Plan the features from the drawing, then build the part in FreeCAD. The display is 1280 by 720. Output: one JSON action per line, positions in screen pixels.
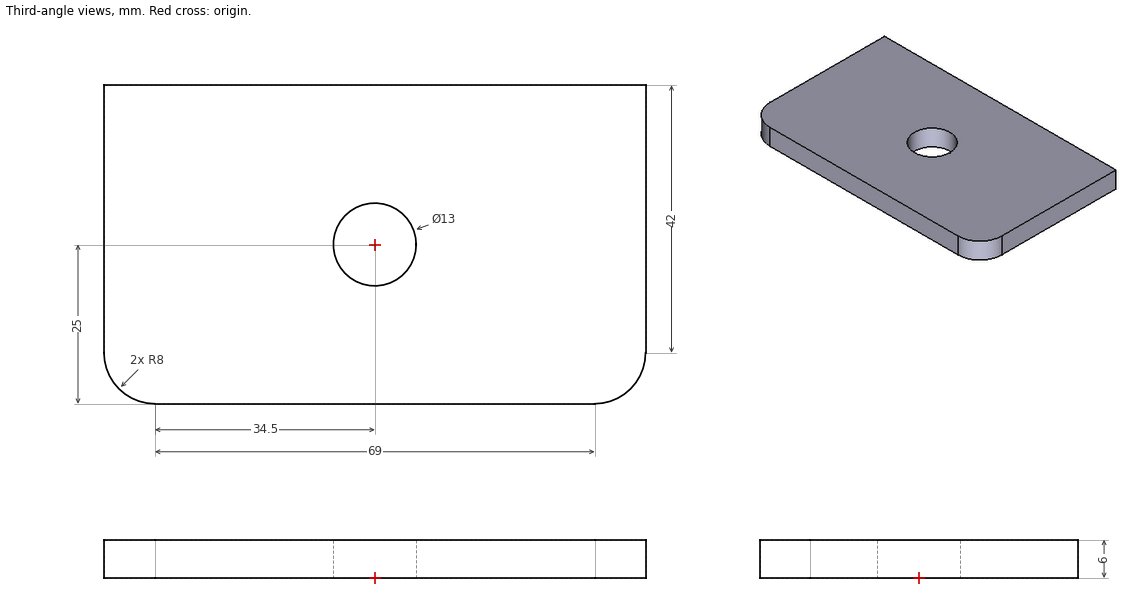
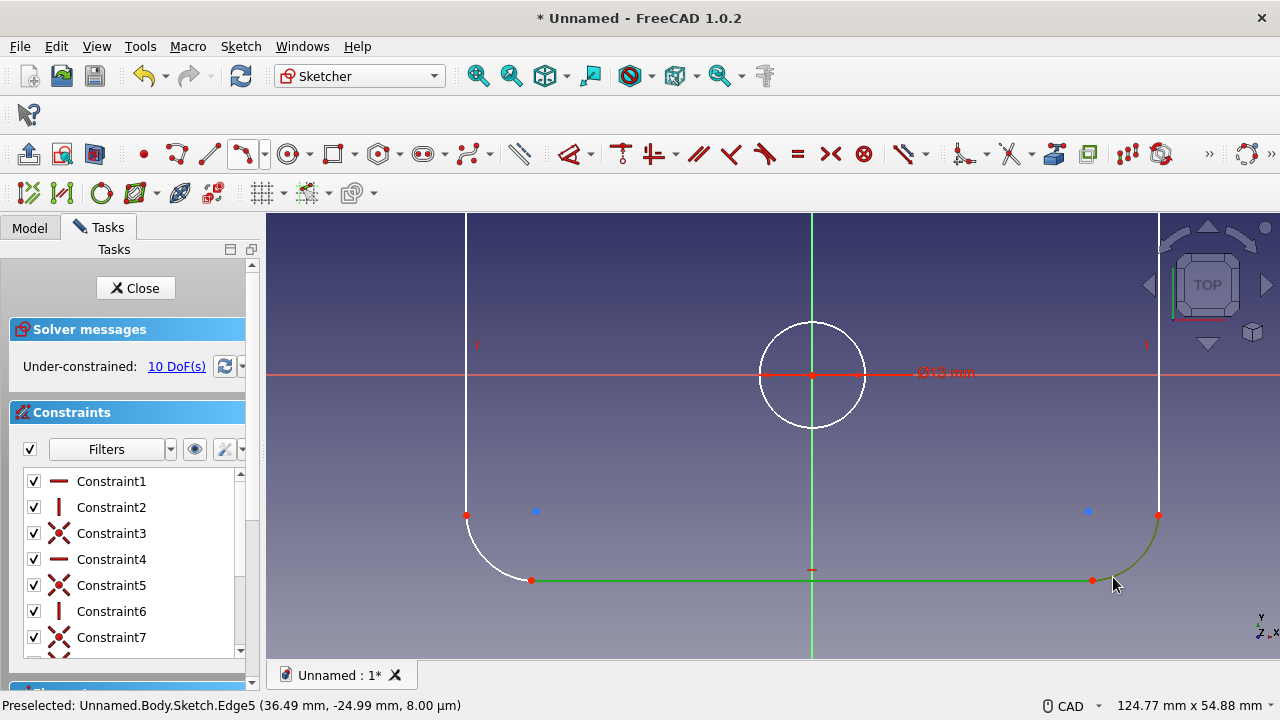
{"action": "left_click", "coordinate": [765, 154]}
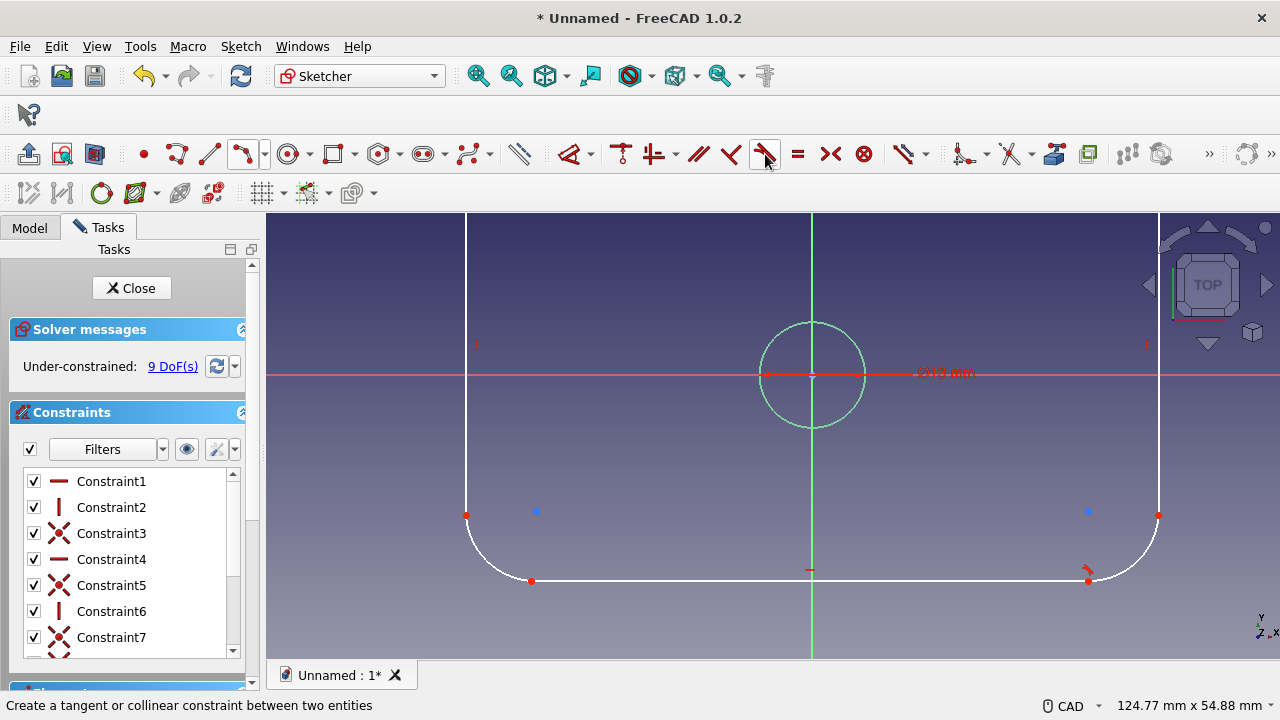
{"action": "left_click", "coordinate": [699, 581]}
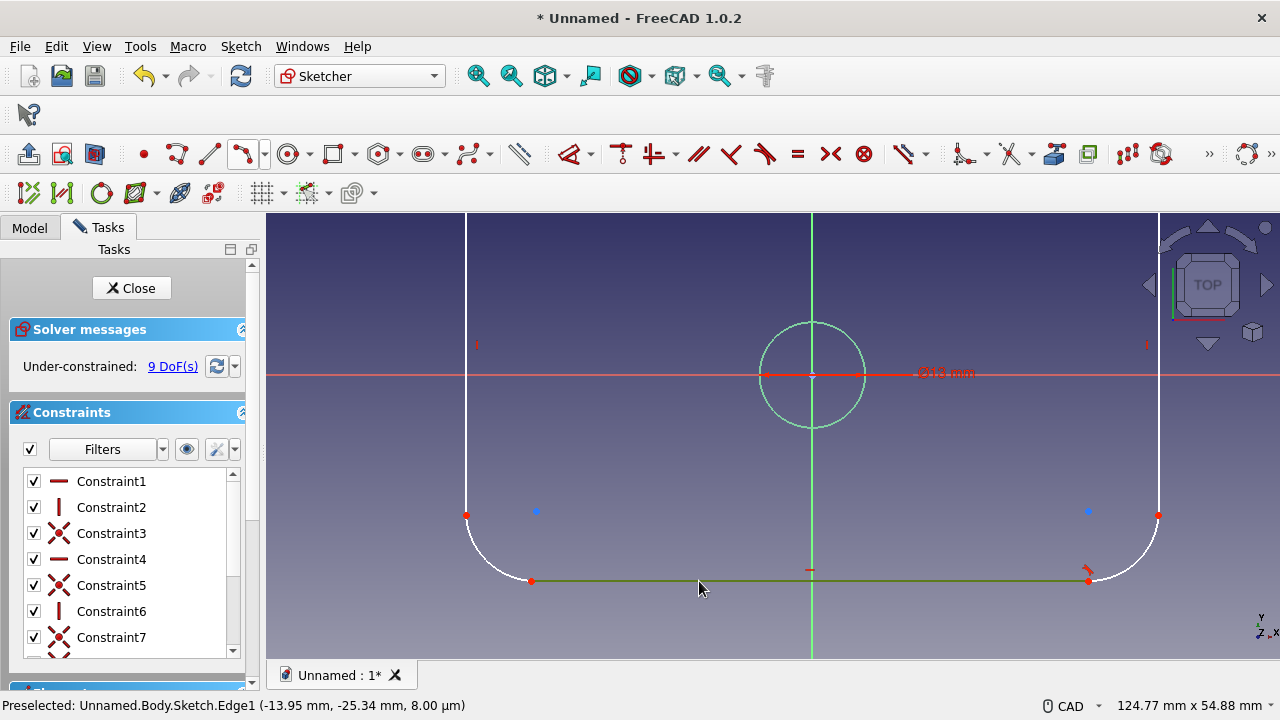
{"action": "left_click", "coordinate": [474, 544]}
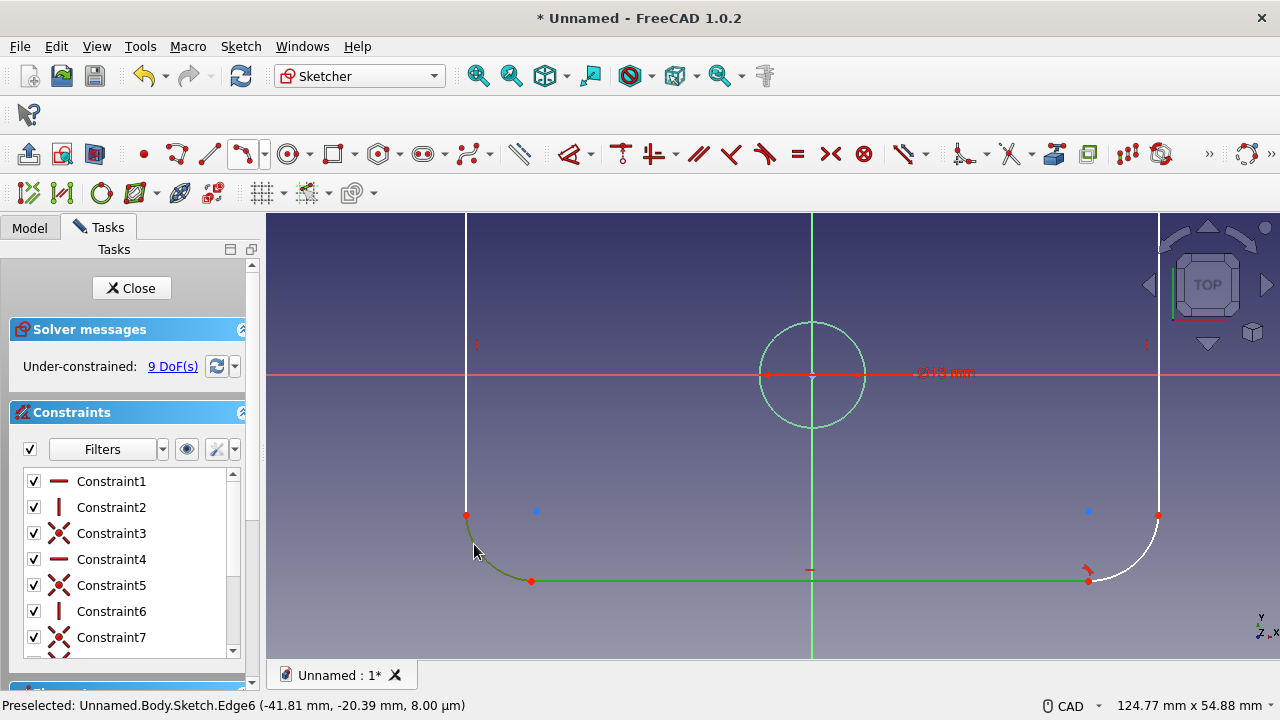
{"action": "left_click", "coordinate": [765, 154]}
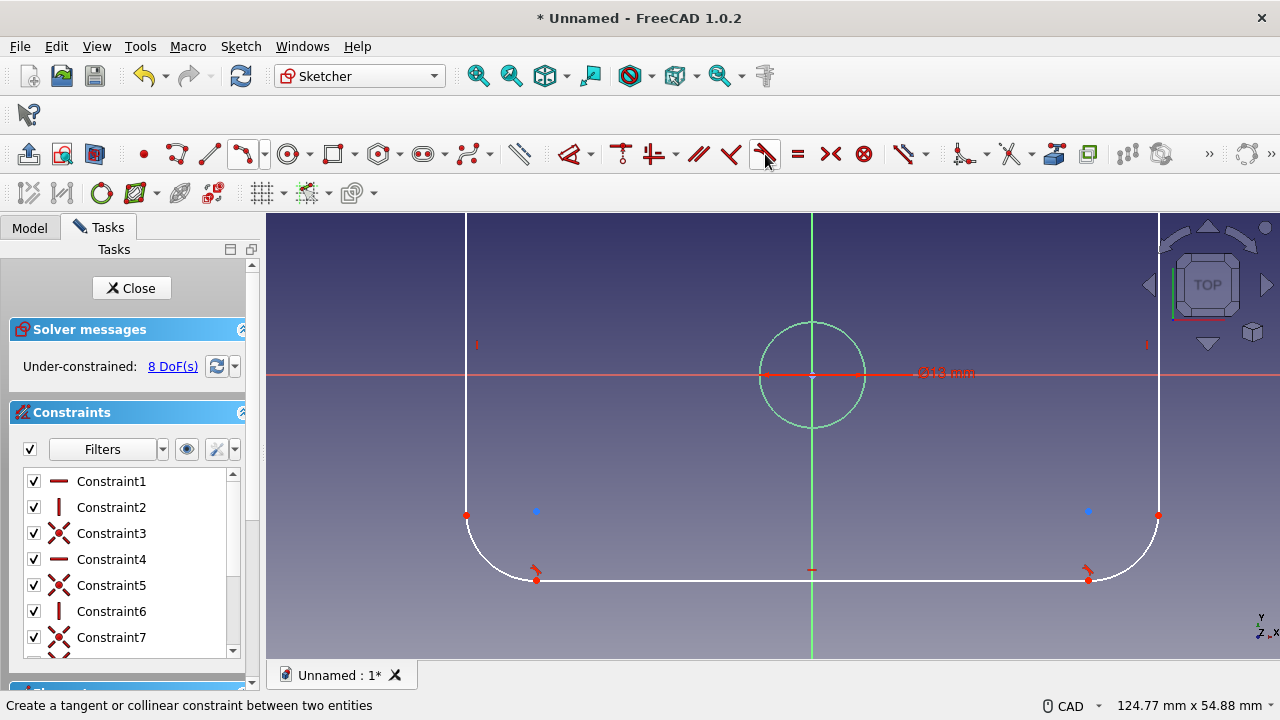
{"action": "scroll", "coordinate": [485, 560], "scroll_direction": "down", "scroll_amount": 2}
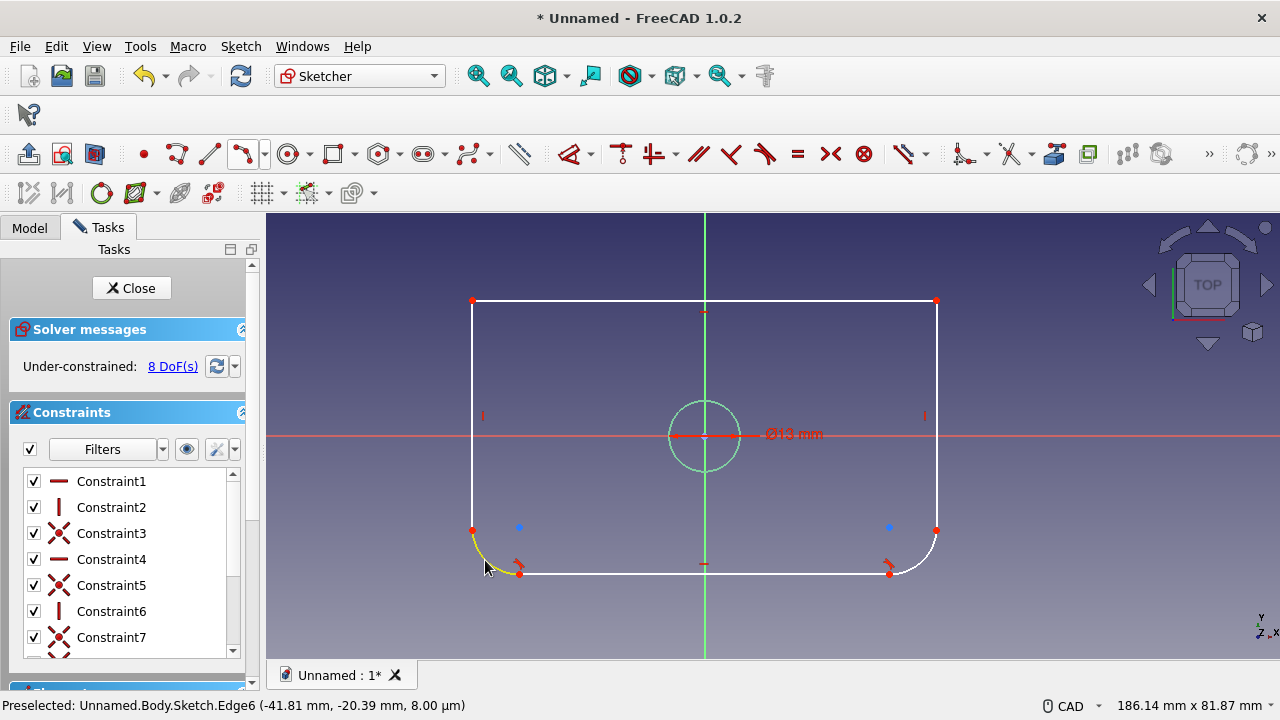
{"action": "left_click", "coordinate": [937, 461]}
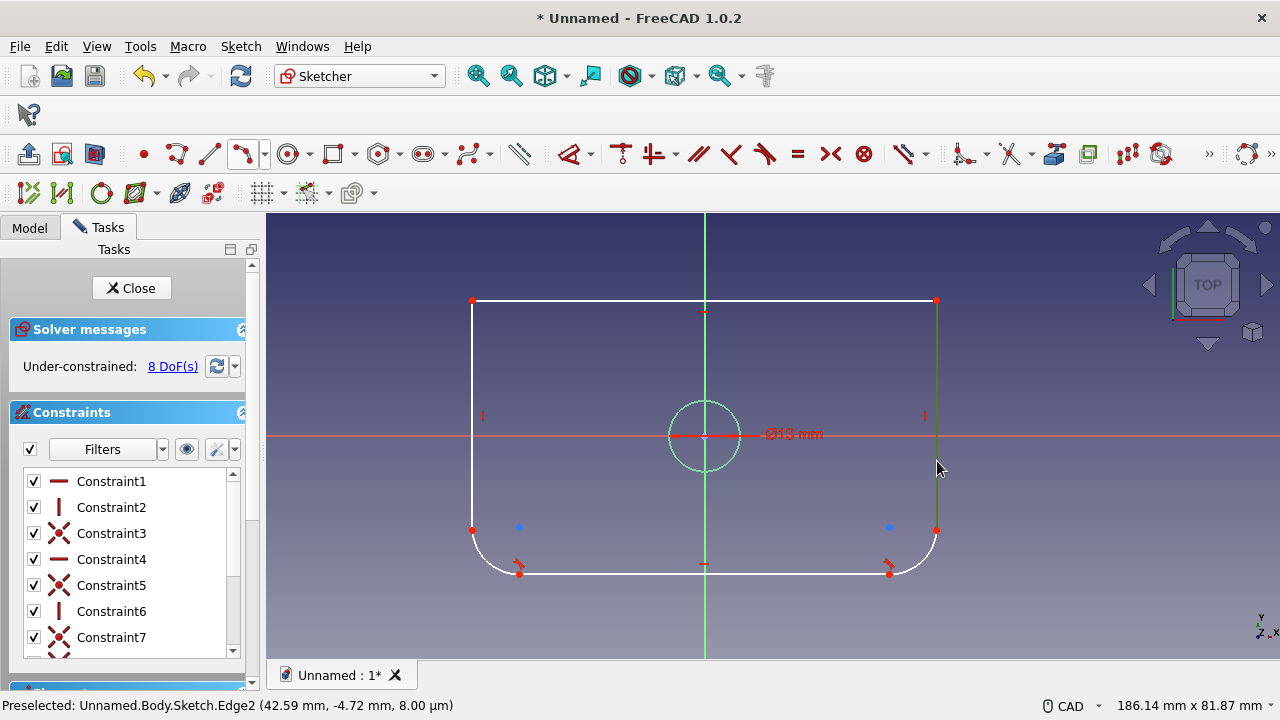
{"action": "left_click", "coordinate": [910, 570]}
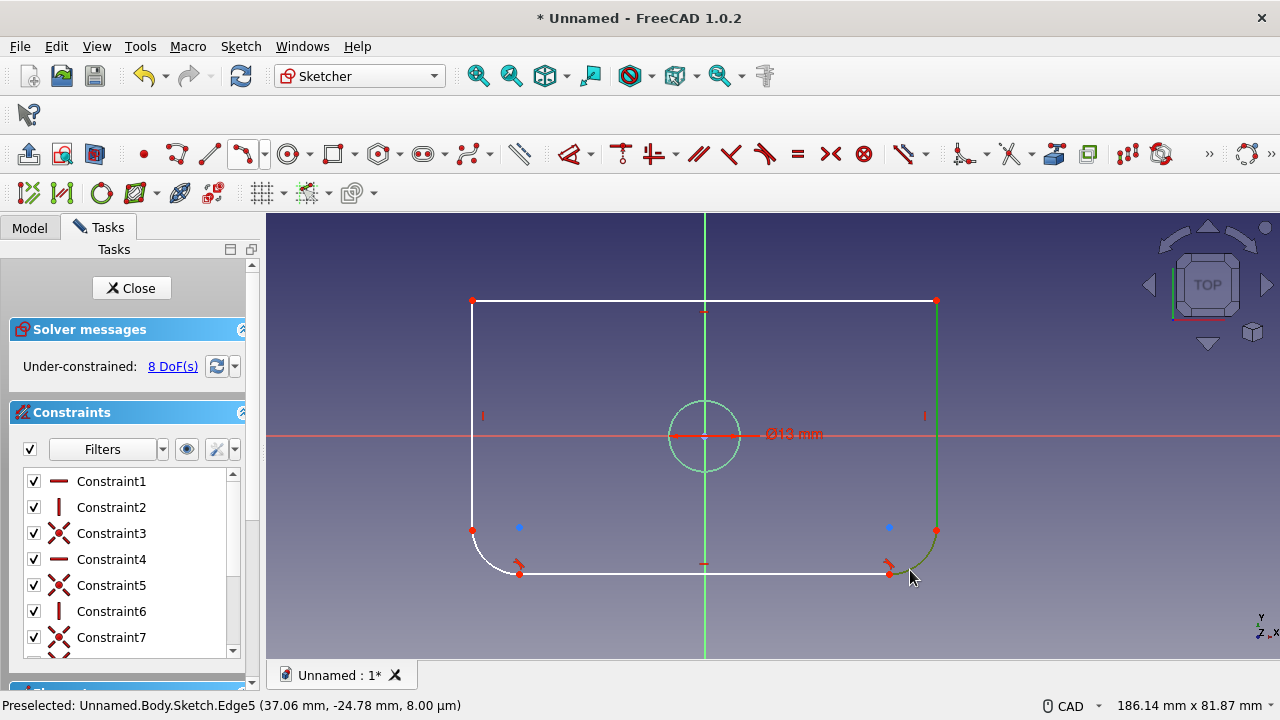
{"action": "left_click", "coordinate": [765, 154]}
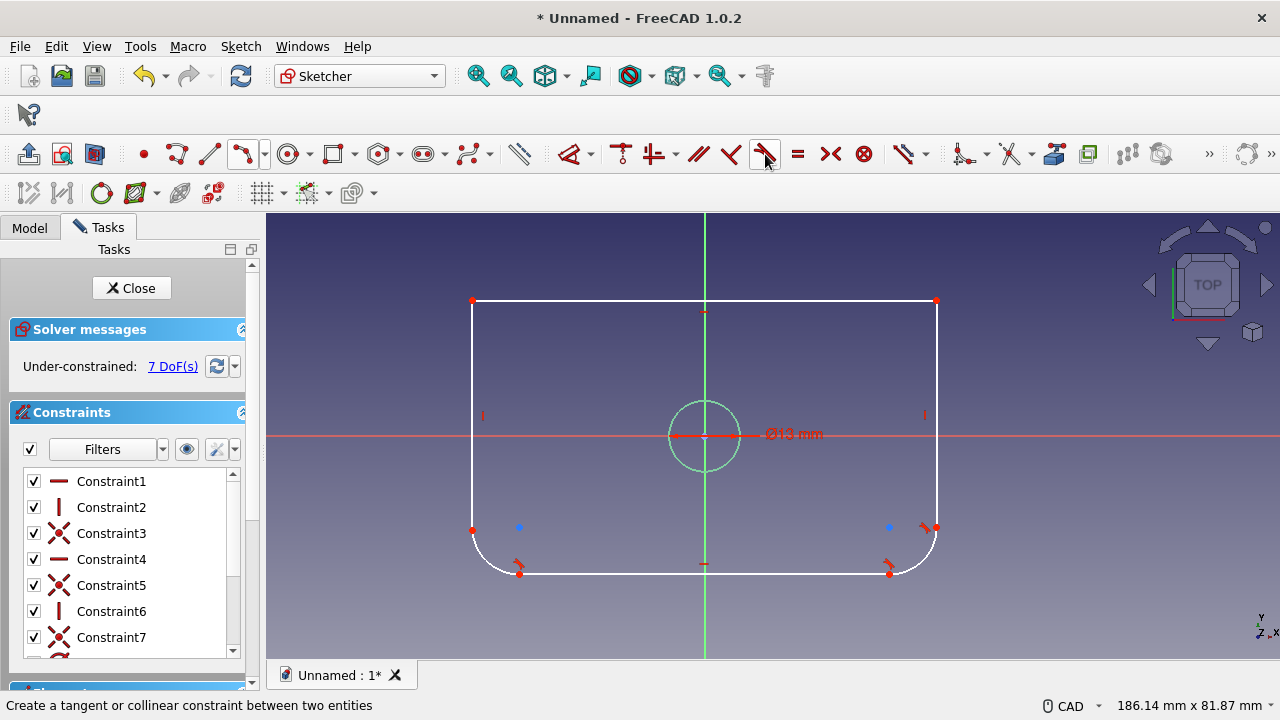
{"action": "left_click", "coordinate": [472, 370]}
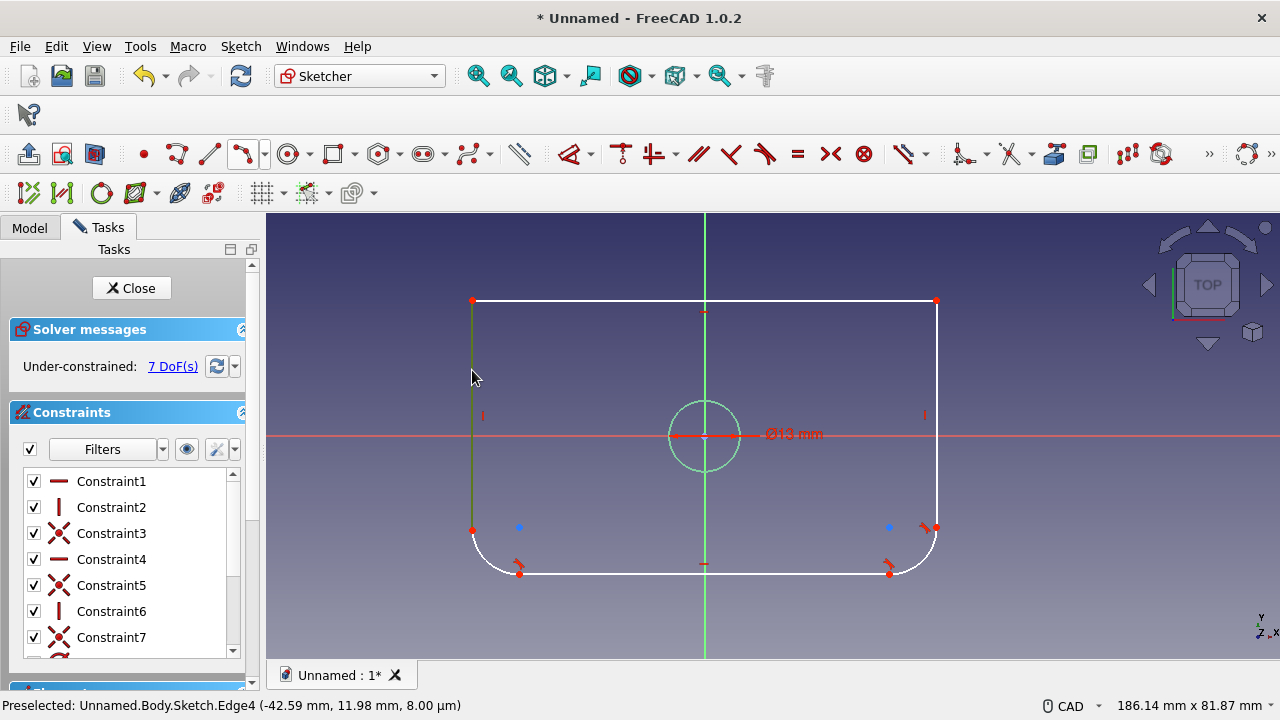
{"action": "left_click", "coordinate": [478, 551]}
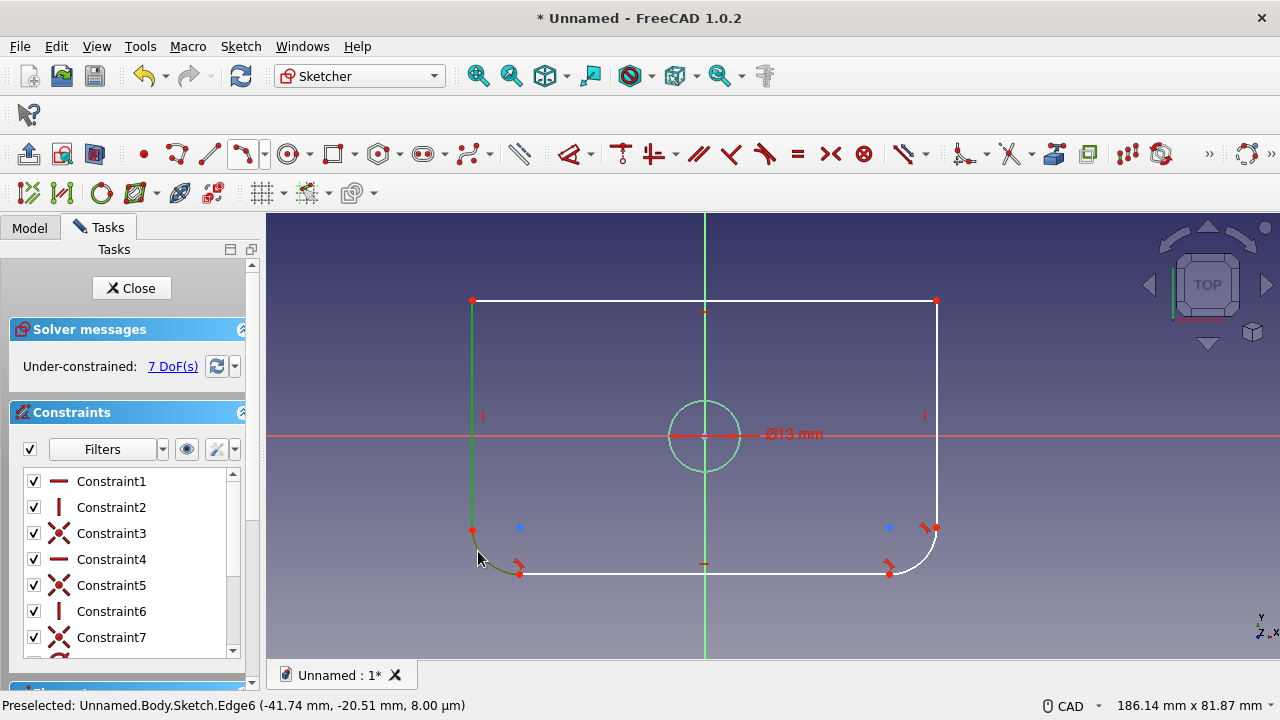
{"action": "left_click", "coordinate": [765, 154]}